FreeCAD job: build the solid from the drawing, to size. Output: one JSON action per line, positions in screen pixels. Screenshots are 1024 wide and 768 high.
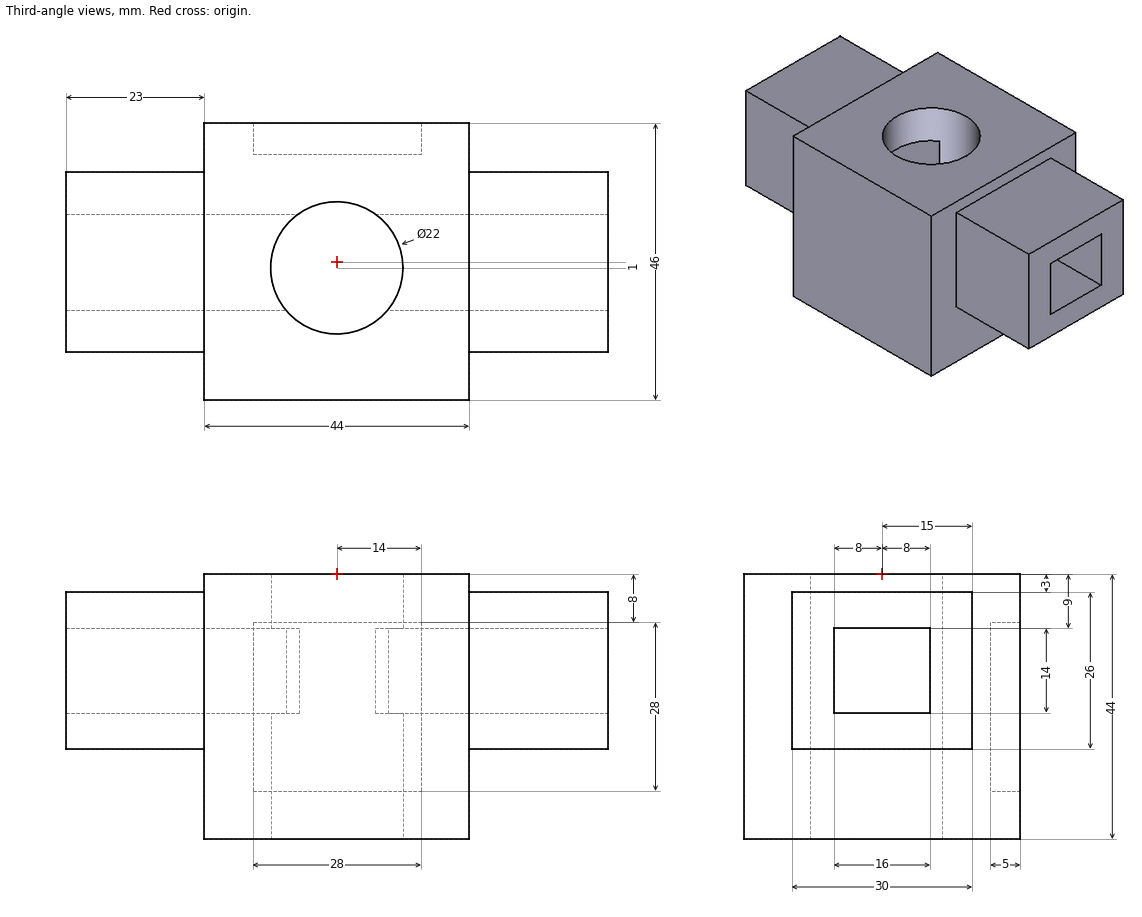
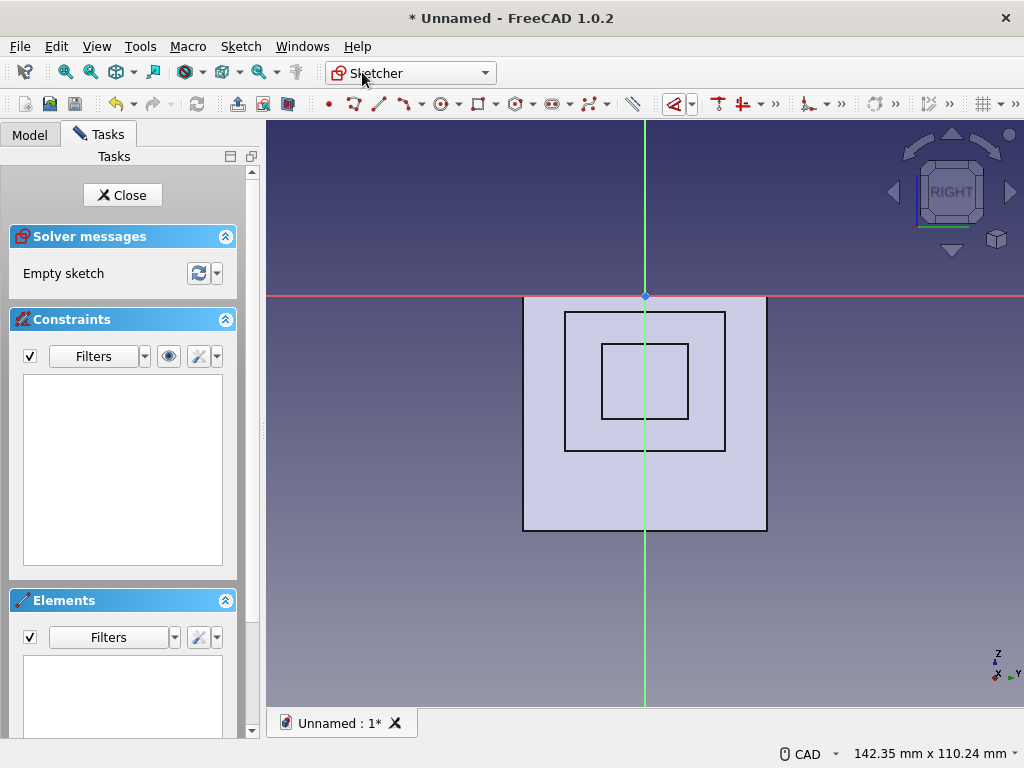
{"action": "scroll", "coordinate": [675, 333], "scroll_direction": "up", "scroll_amount": 6}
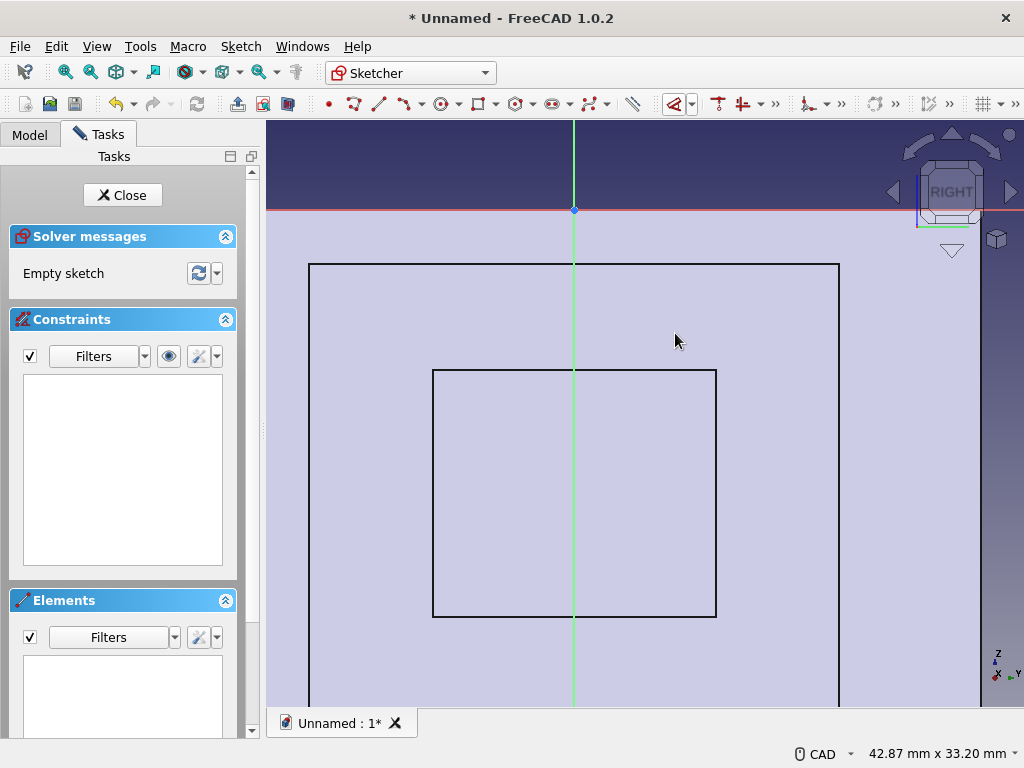
{"action": "key", "text": "g r"}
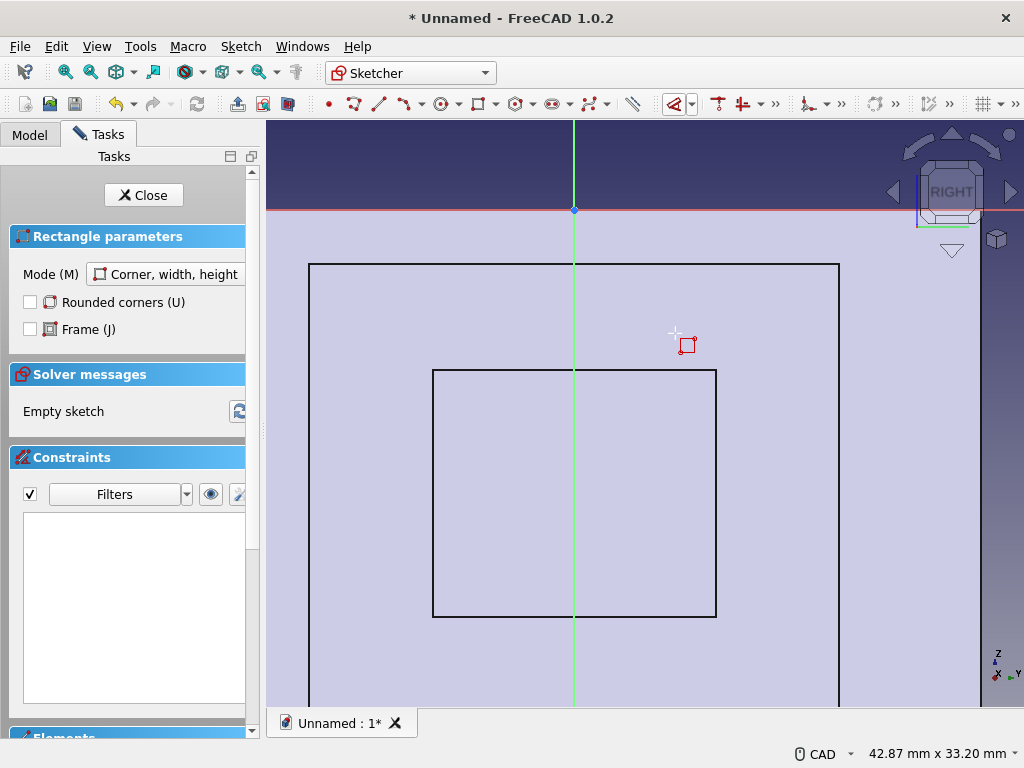
{"action": "left_click", "coordinate": [433, 370]}
{"action": "left_click", "coordinate": [716, 617]}
{"action": "key", "text": "Escape"}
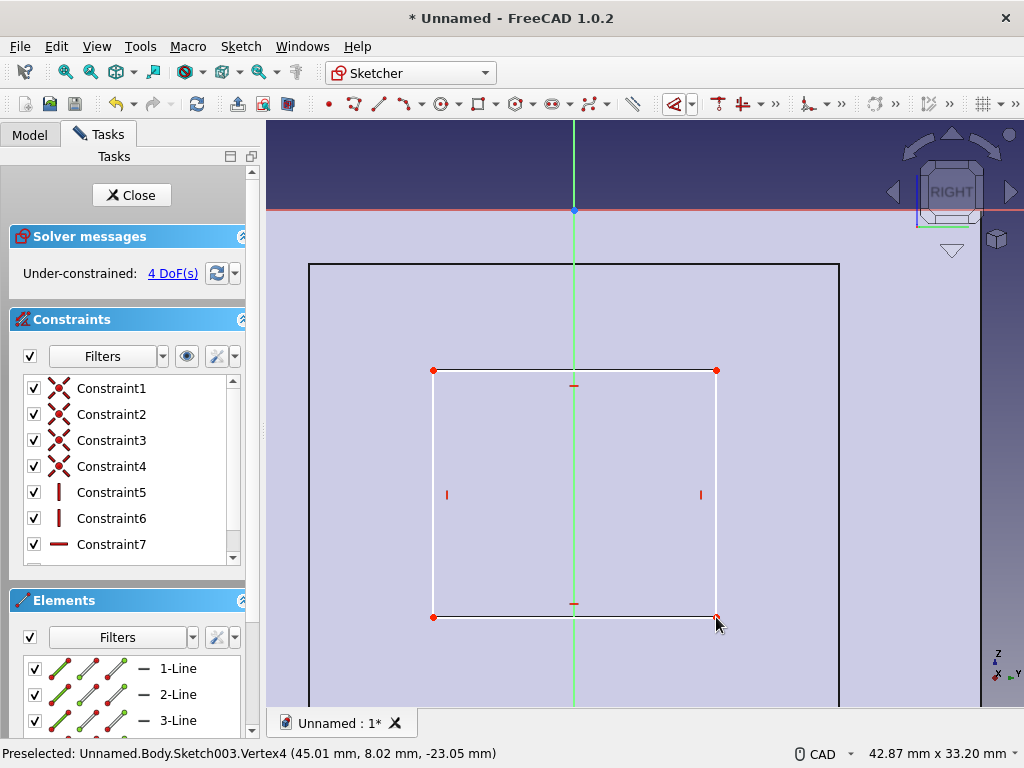
{"action": "left_click", "coordinate": [433, 445]}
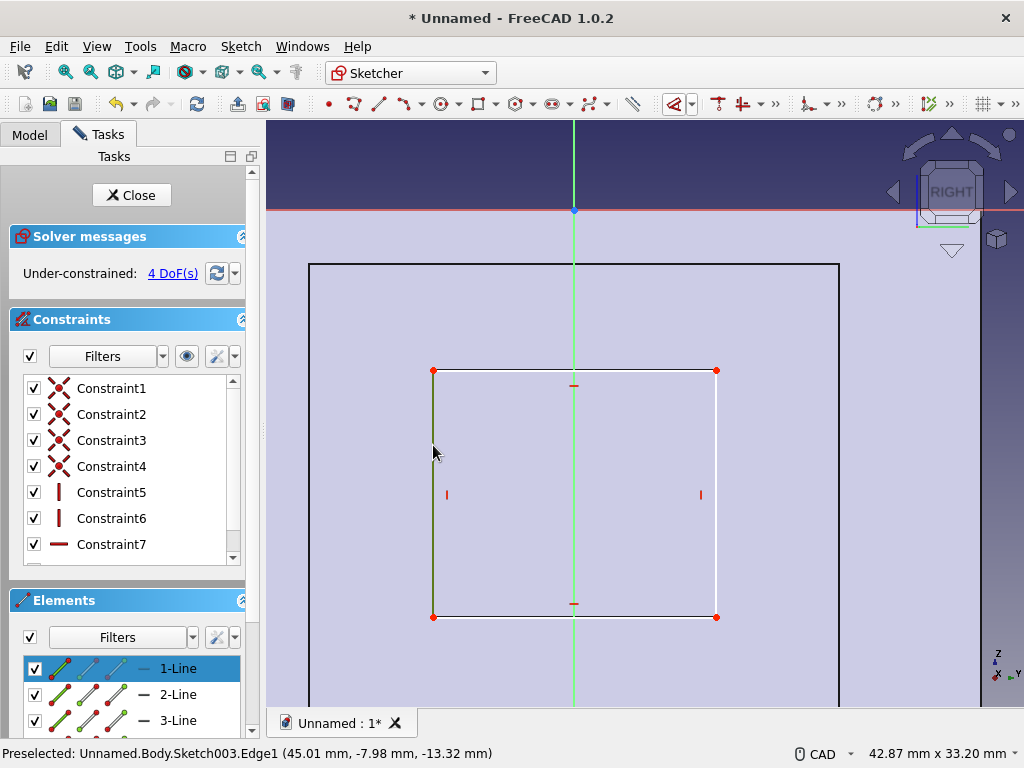
{"action": "left_click", "coordinate": [692, 104]}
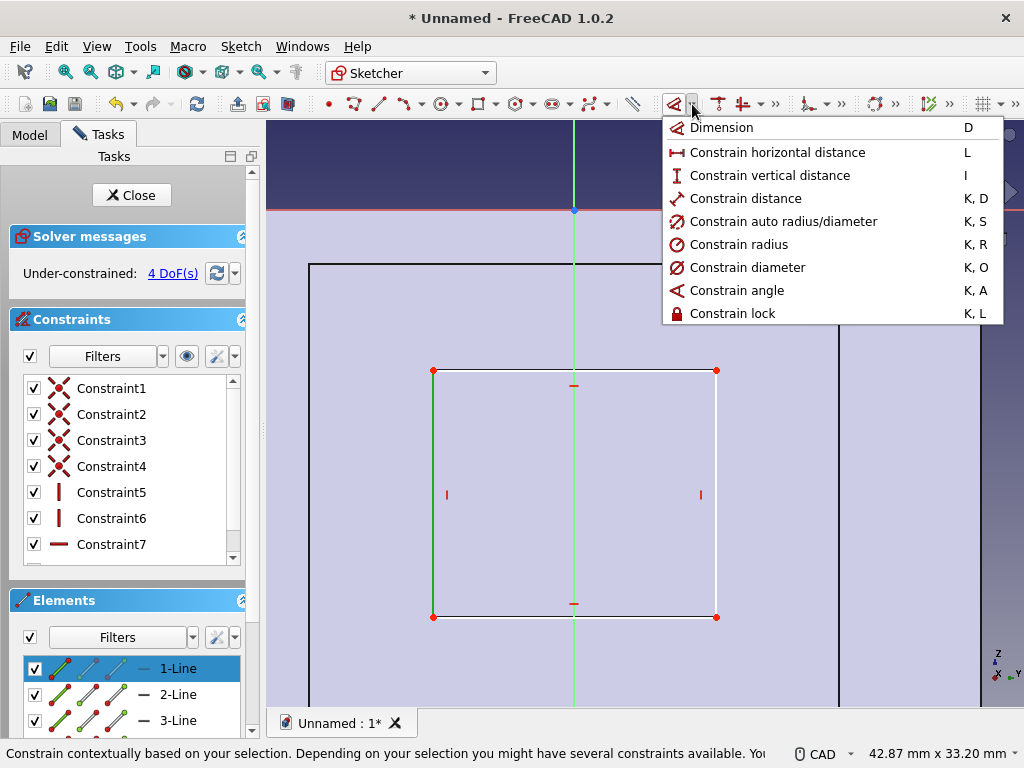
{"action": "left_click", "coordinate": [833, 176]}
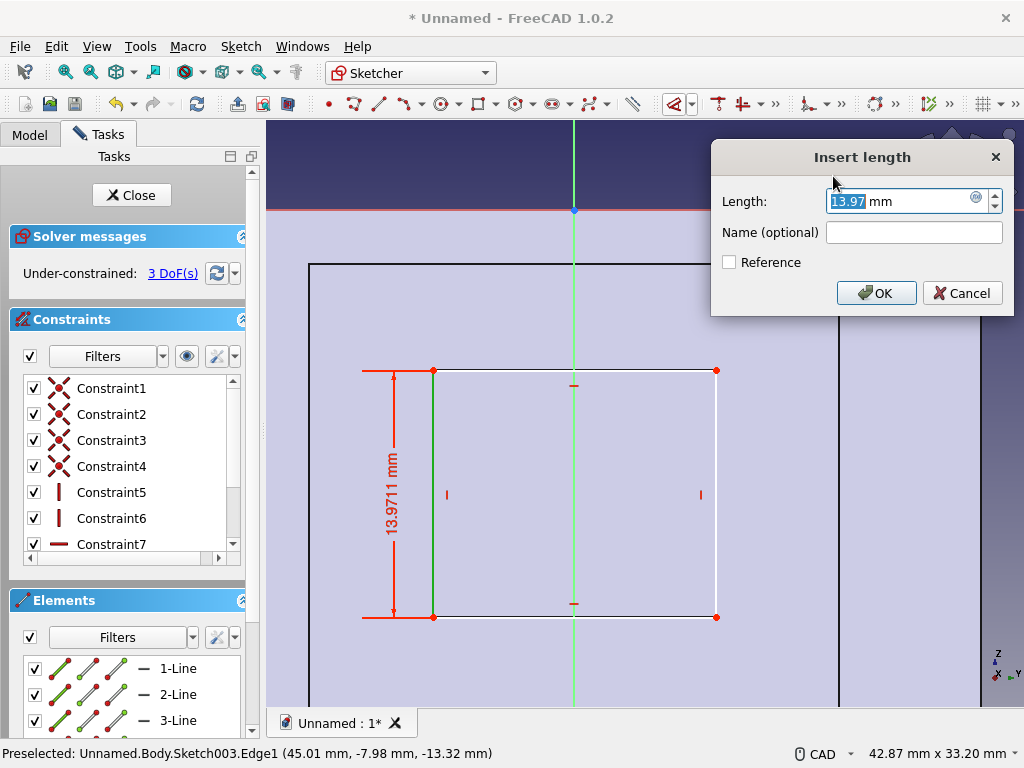
{"action": "type", "text": "14"}
{"action": "key", "text": "Return"}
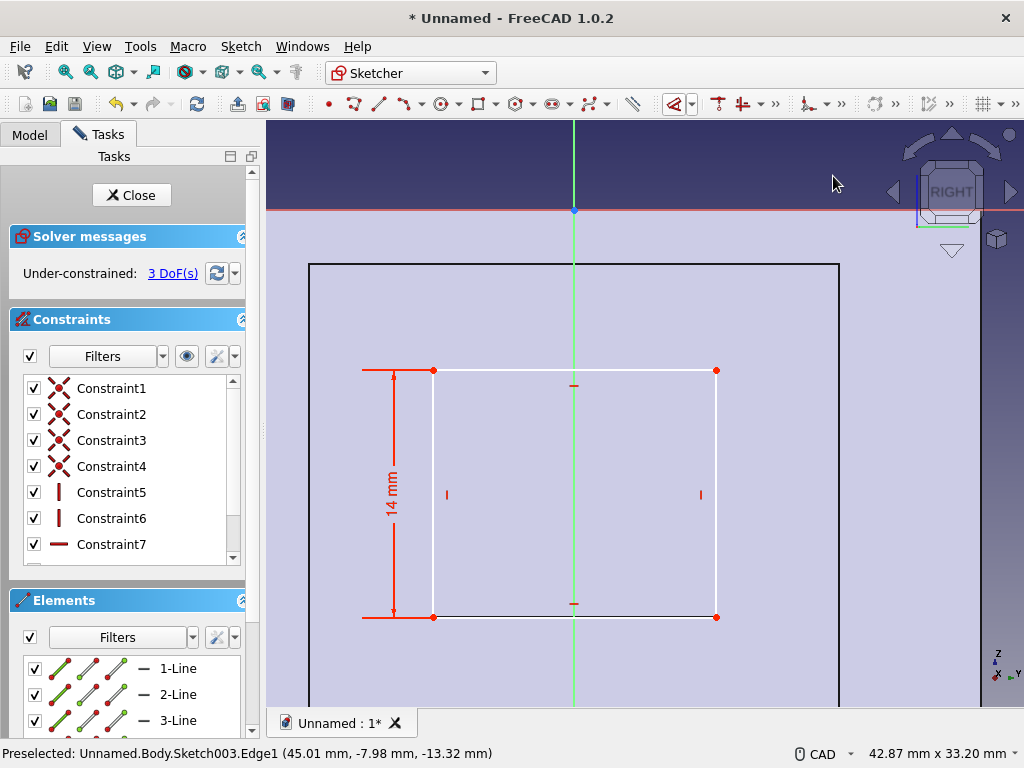
{"action": "left_click", "coordinate": [518, 618]}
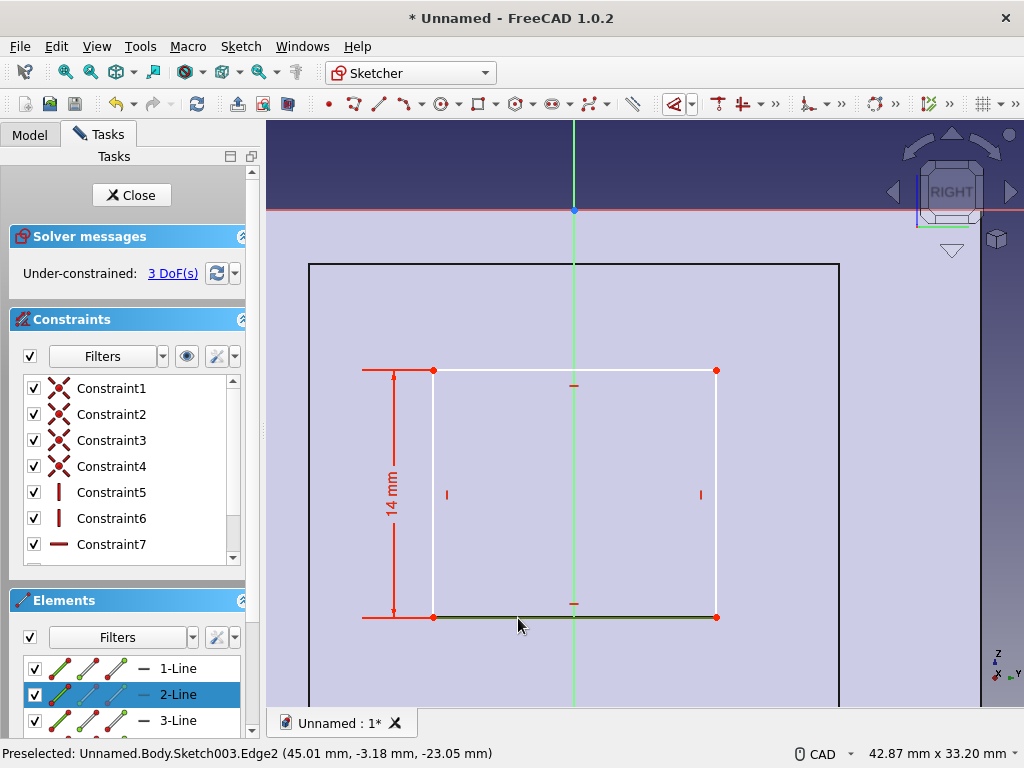
{"action": "key", "text": "l"}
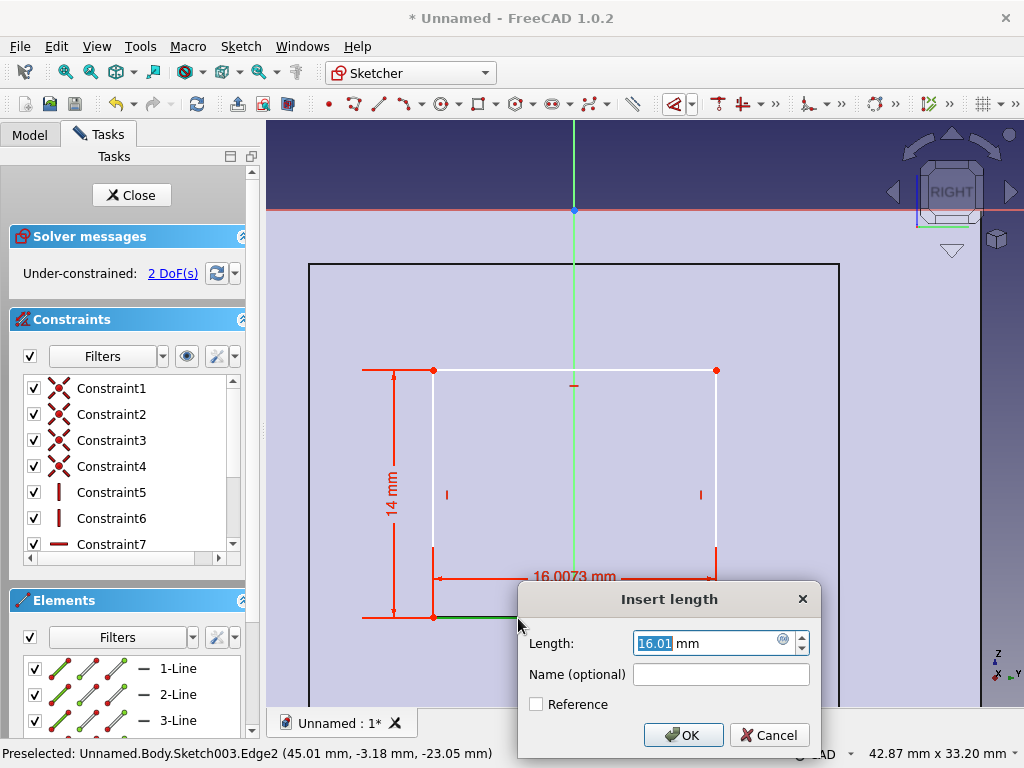
{"action": "type", "text": "16"}
{"action": "key", "text": "Return"}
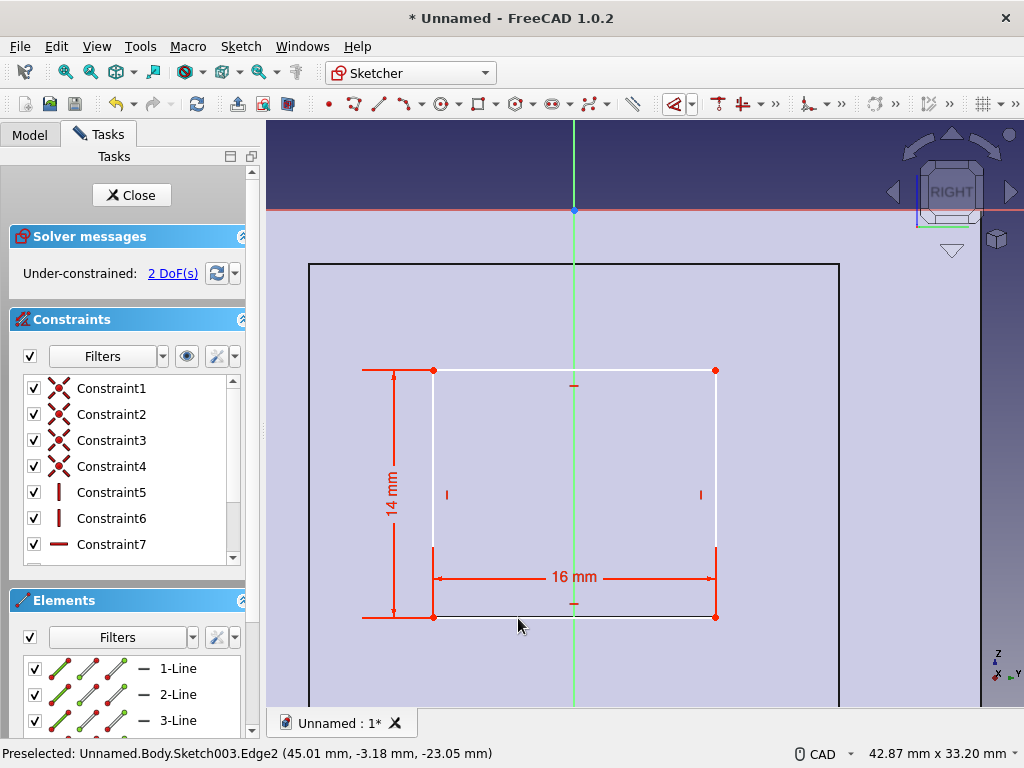
{"action": "left_click", "coordinate": [433, 370]}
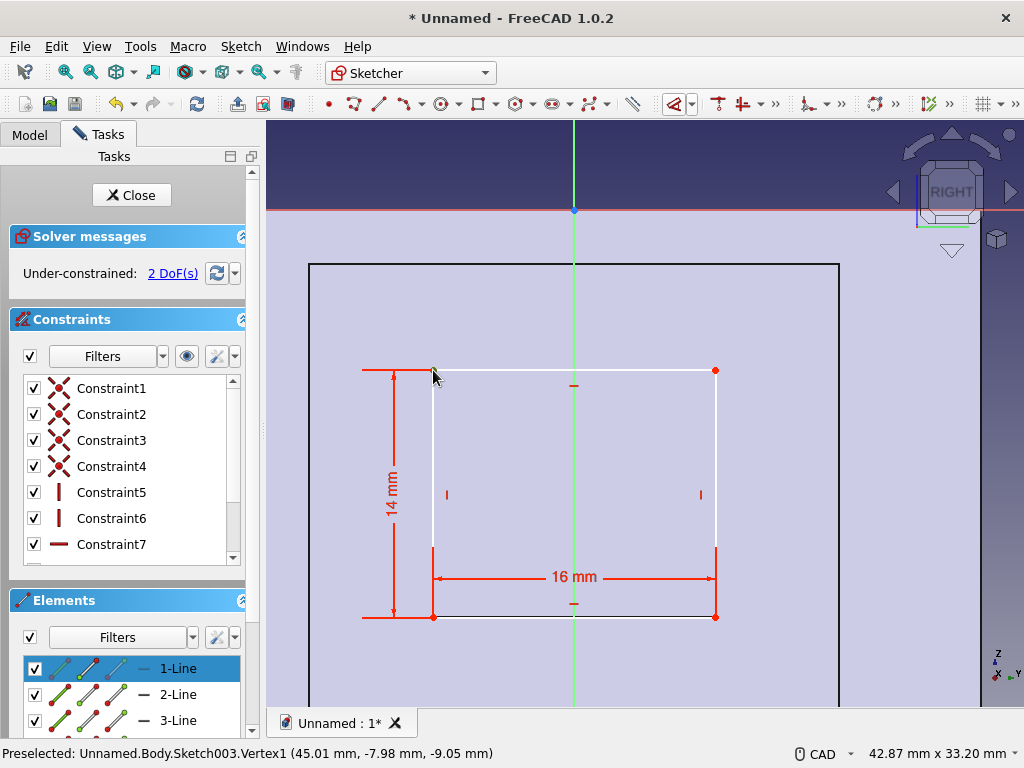
{"action": "key", "text": "l"}